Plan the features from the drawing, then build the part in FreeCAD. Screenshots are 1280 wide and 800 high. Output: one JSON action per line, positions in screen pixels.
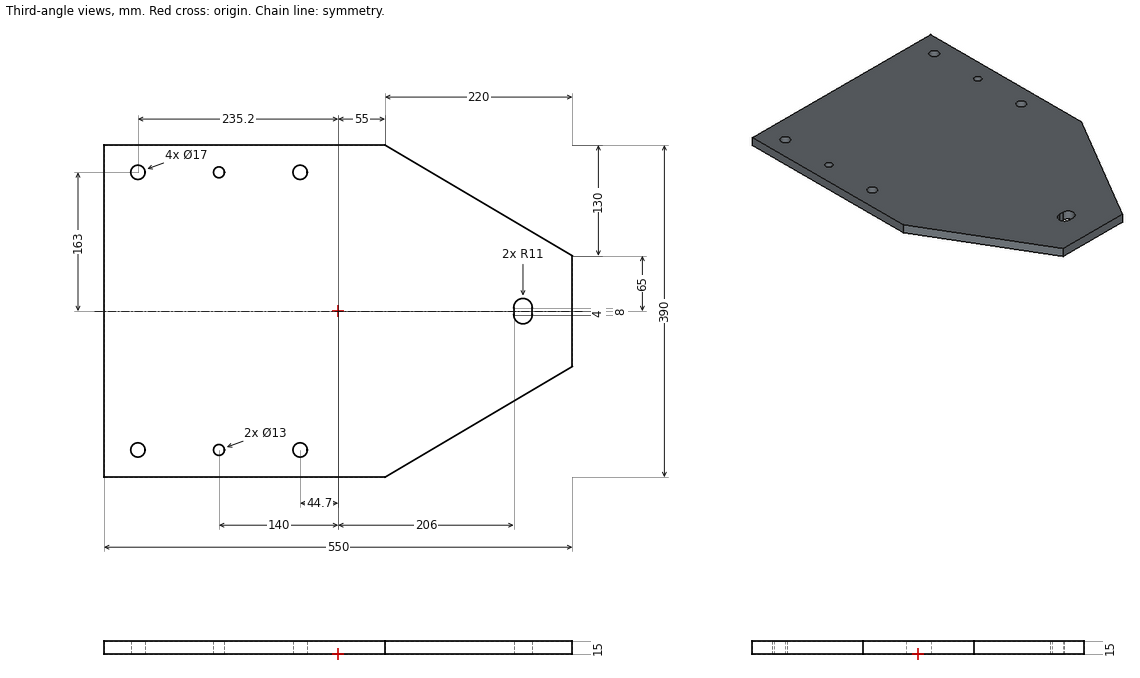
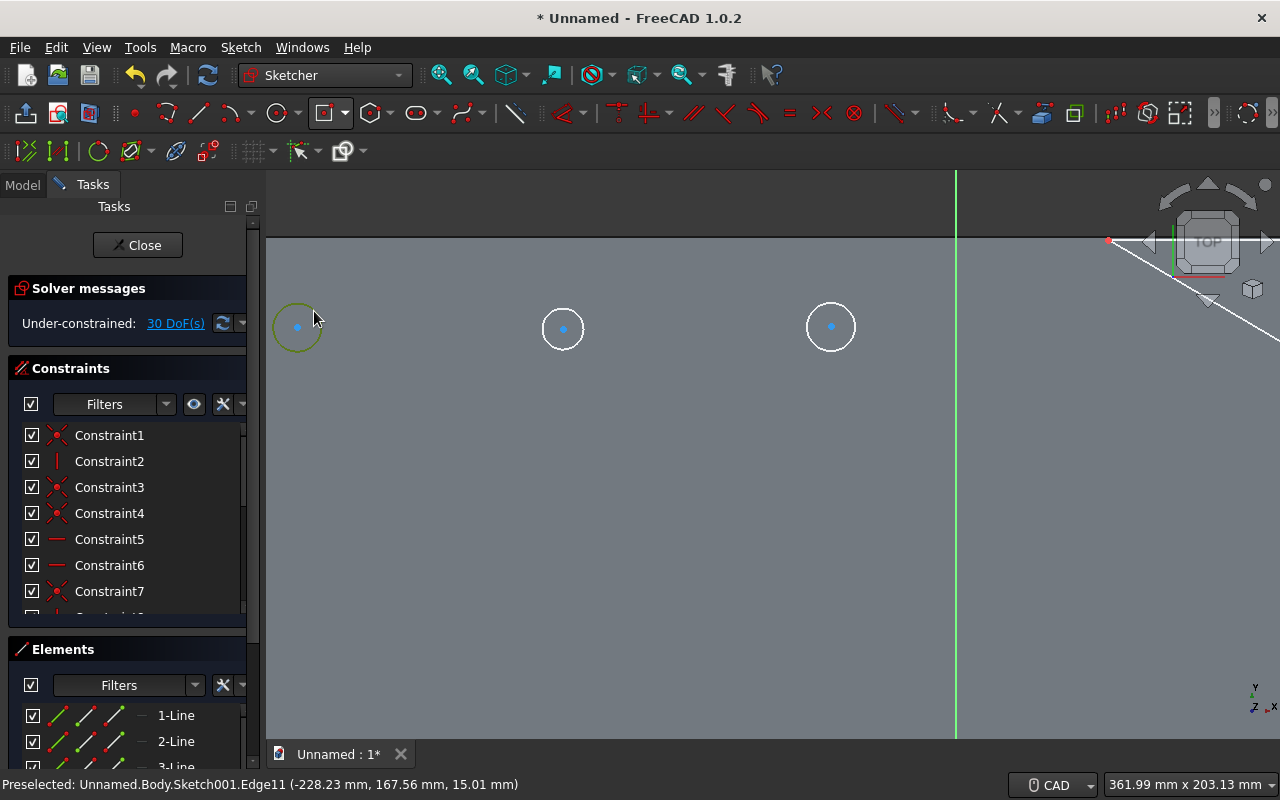
{"action": "scroll", "coordinate": [577, 313], "scroll_direction": "down", "scroll_amount": 6}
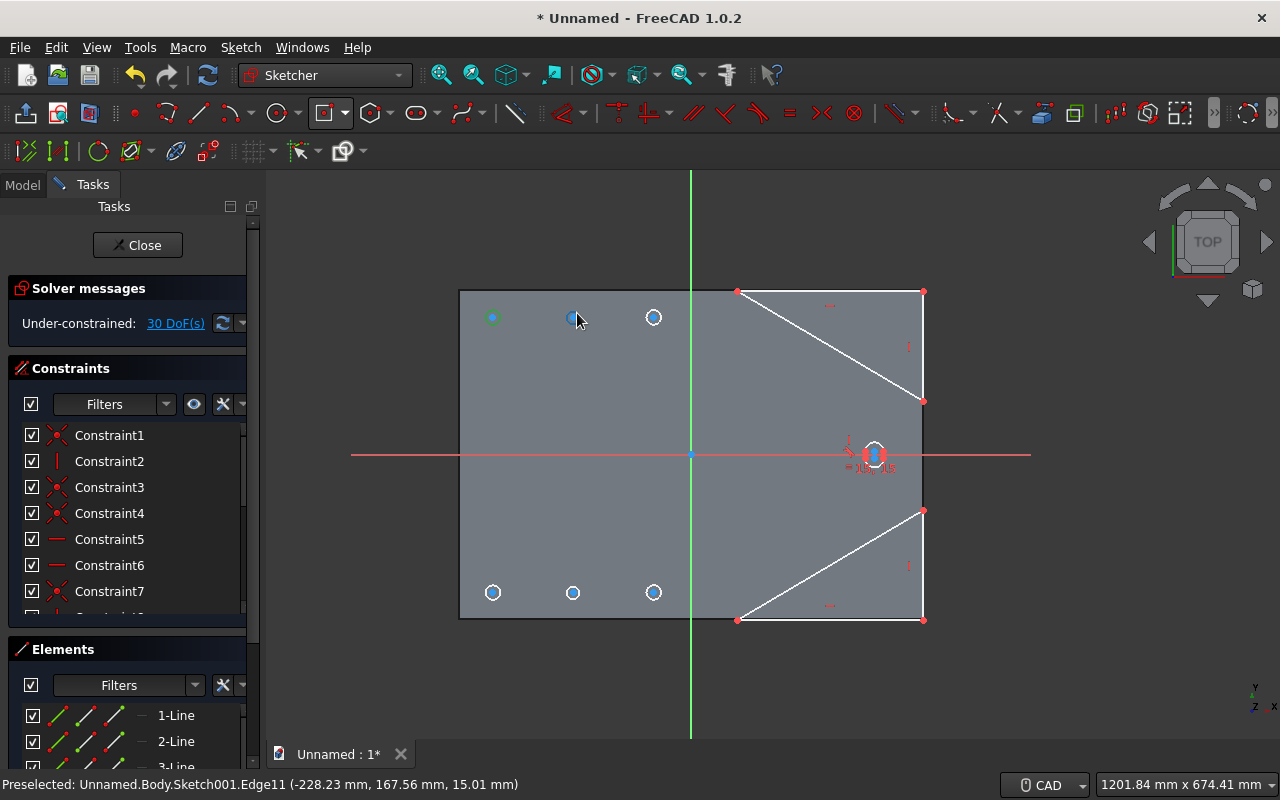
{"action": "scroll", "coordinate": [498, 587], "scroll_direction": "up", "scroll_amount": 4}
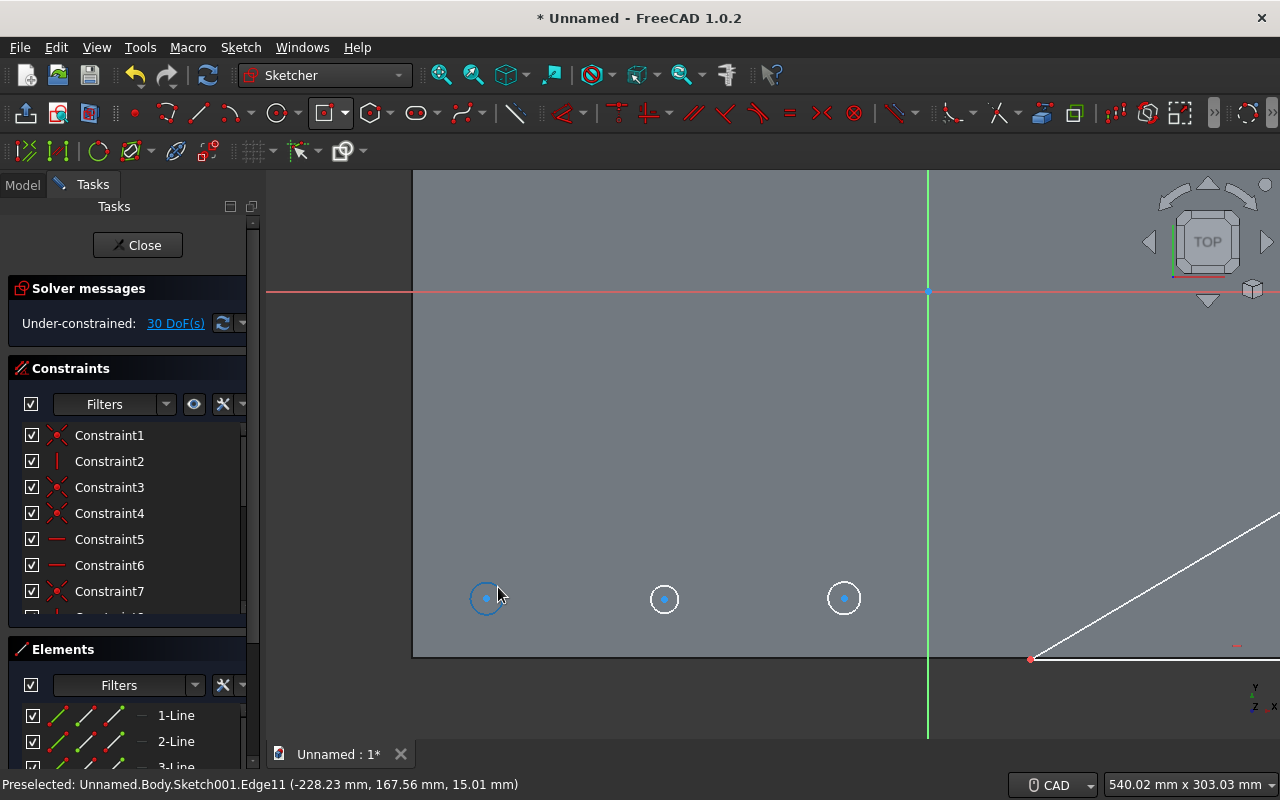
{"action": "left_click", "coordinate": [498, 587]}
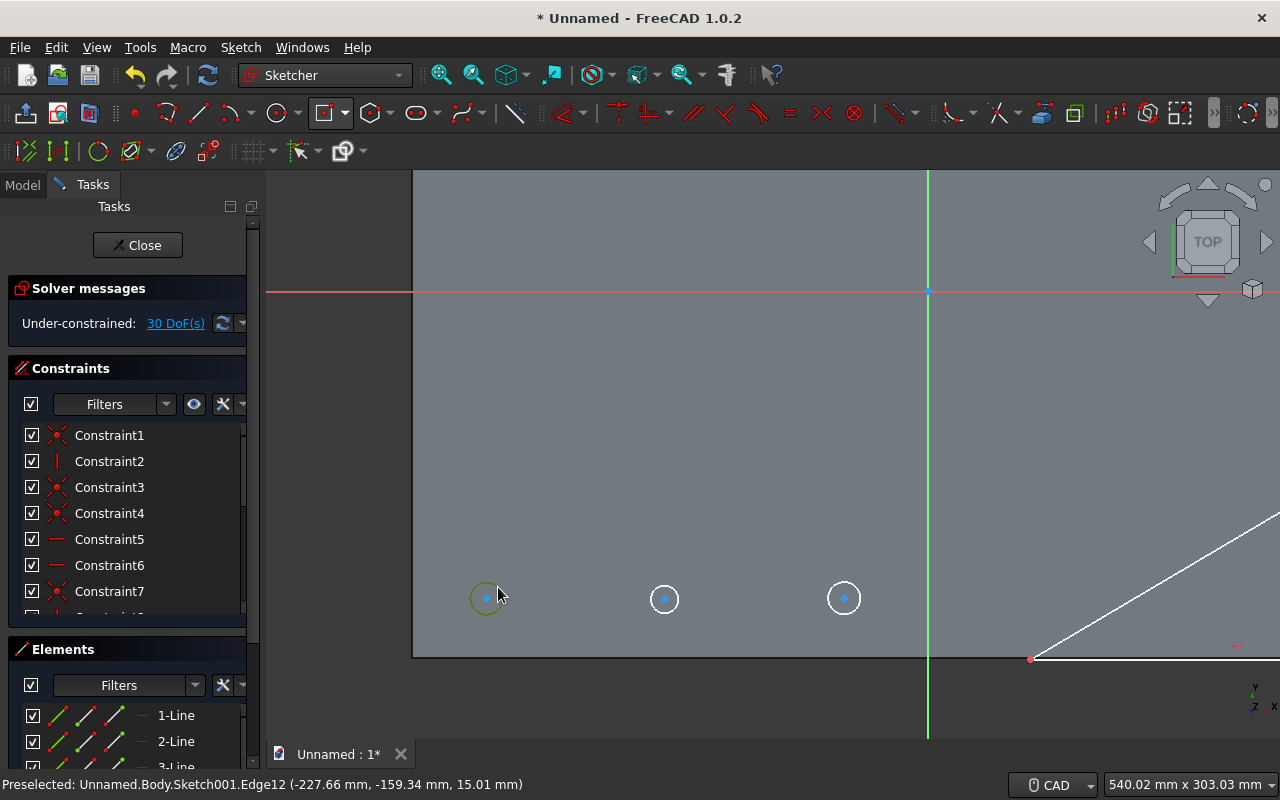
{"action": "left_click", "coordinate": [856, 587]}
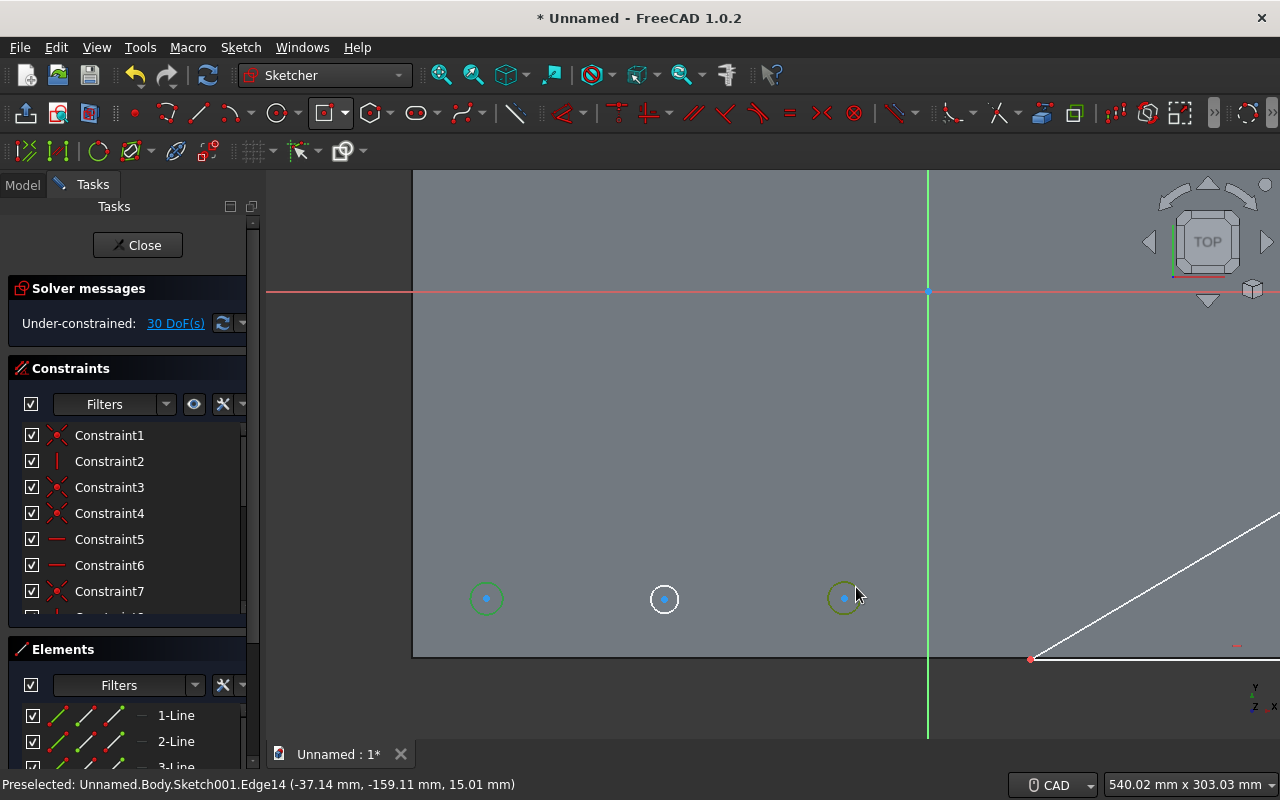
{"action": "scroll", "coordinate": [498, 587], "scroll_direction": "down", "scroll_amount": 4}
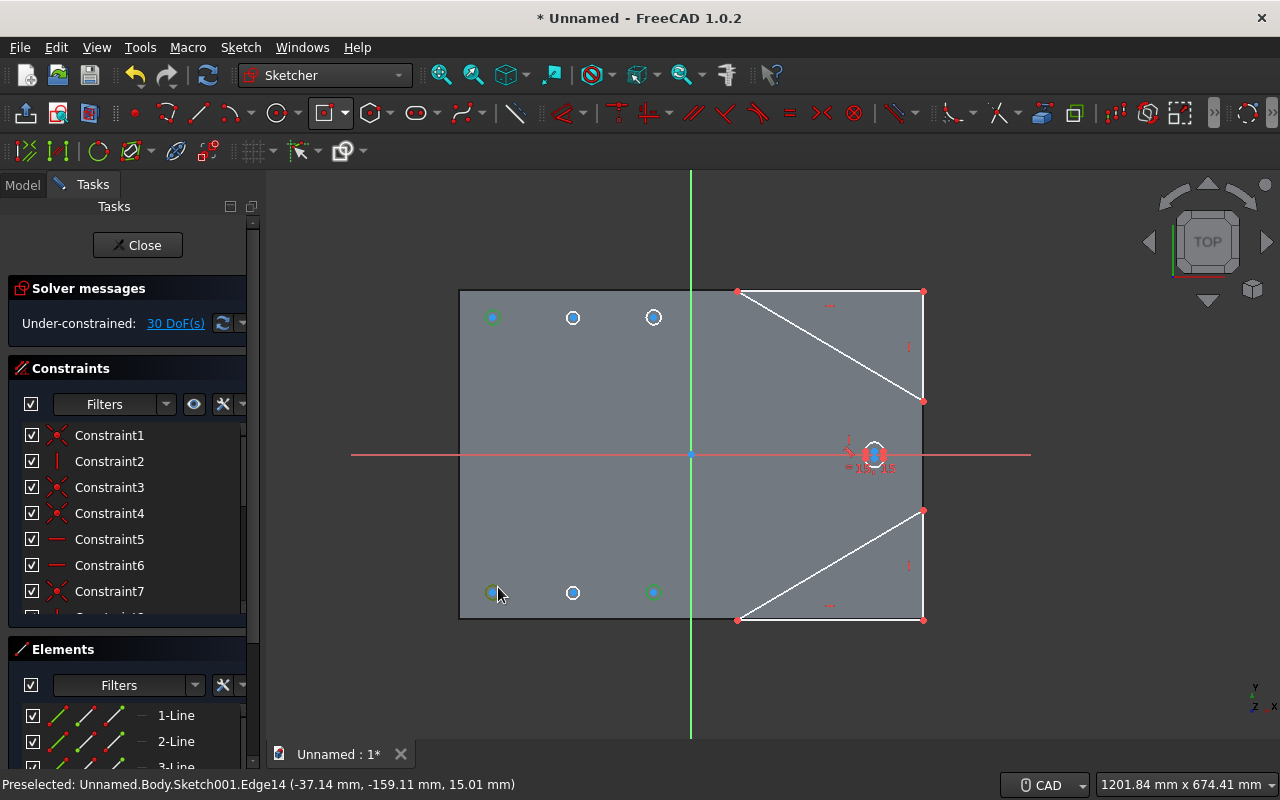
{"action": "scroll", "coordinate": [659, 312], "scroll_direction": "up", "scroll_amount": 4}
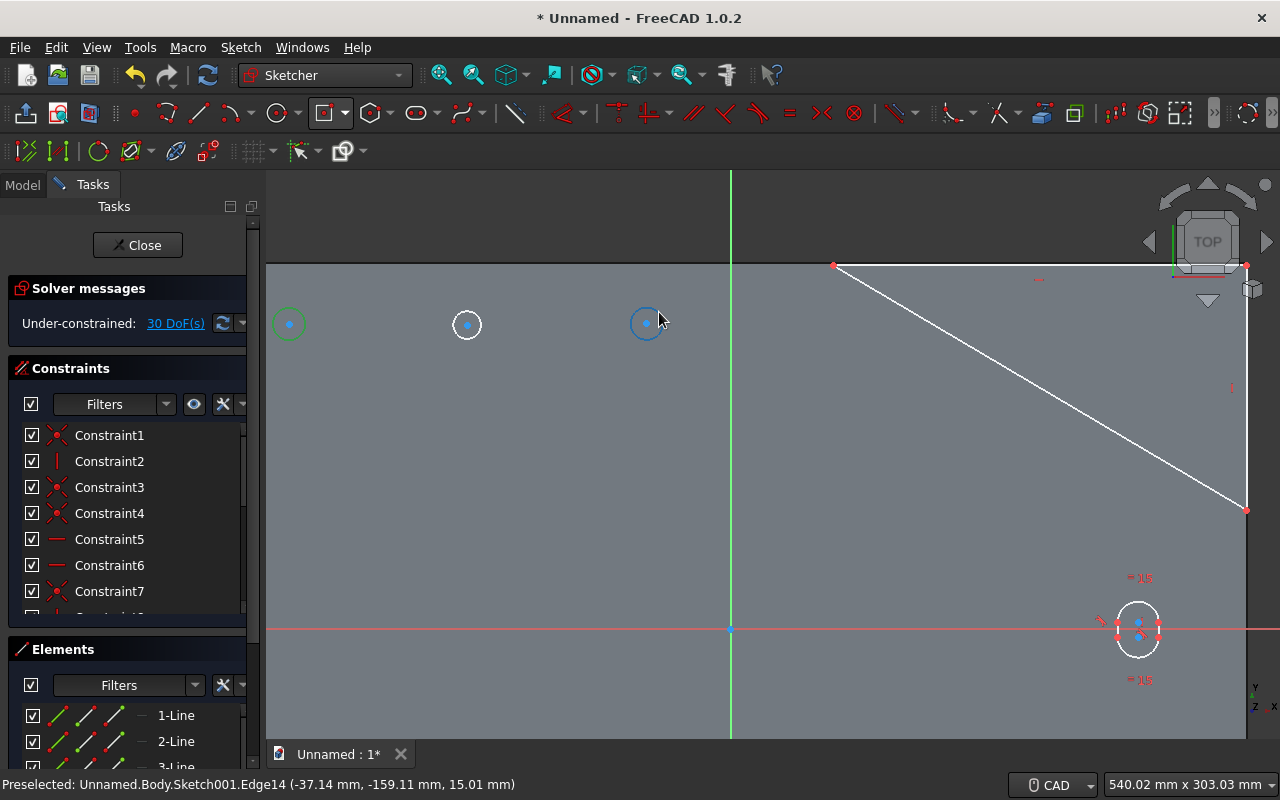
{"action": "left_click", "coordinate": [658, 312]}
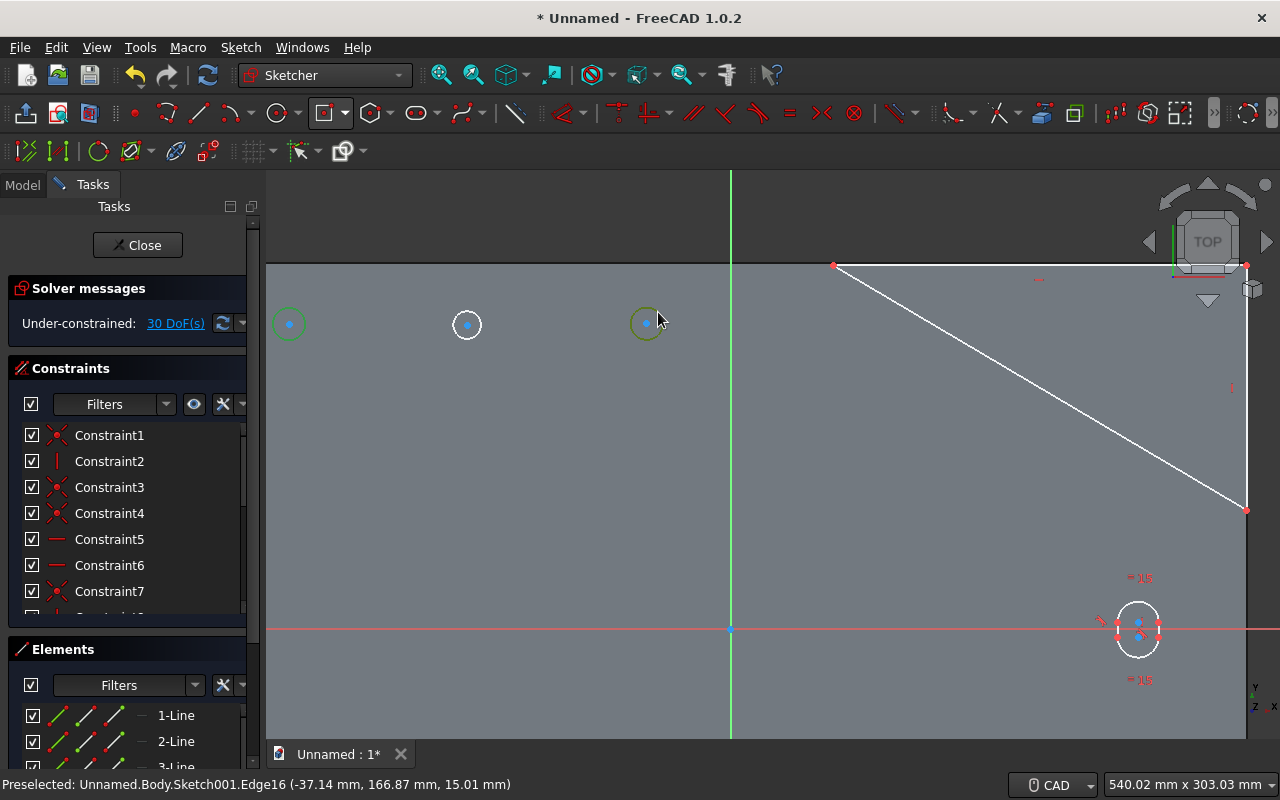
{"action": "left_click", "coordinate": [790, 114]}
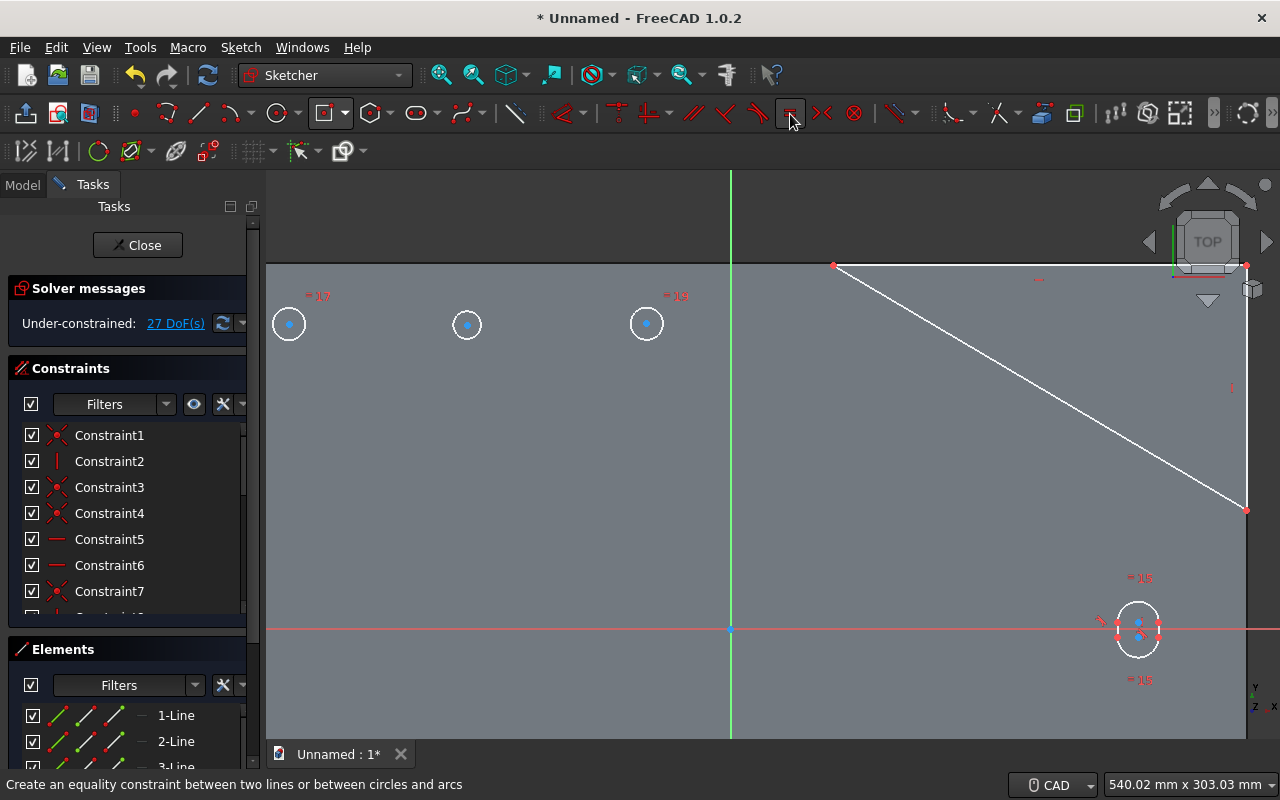
{"action": "scroll", "coordinate": [659, 312], "scroll_direction": "down", "scroll_amount": 4}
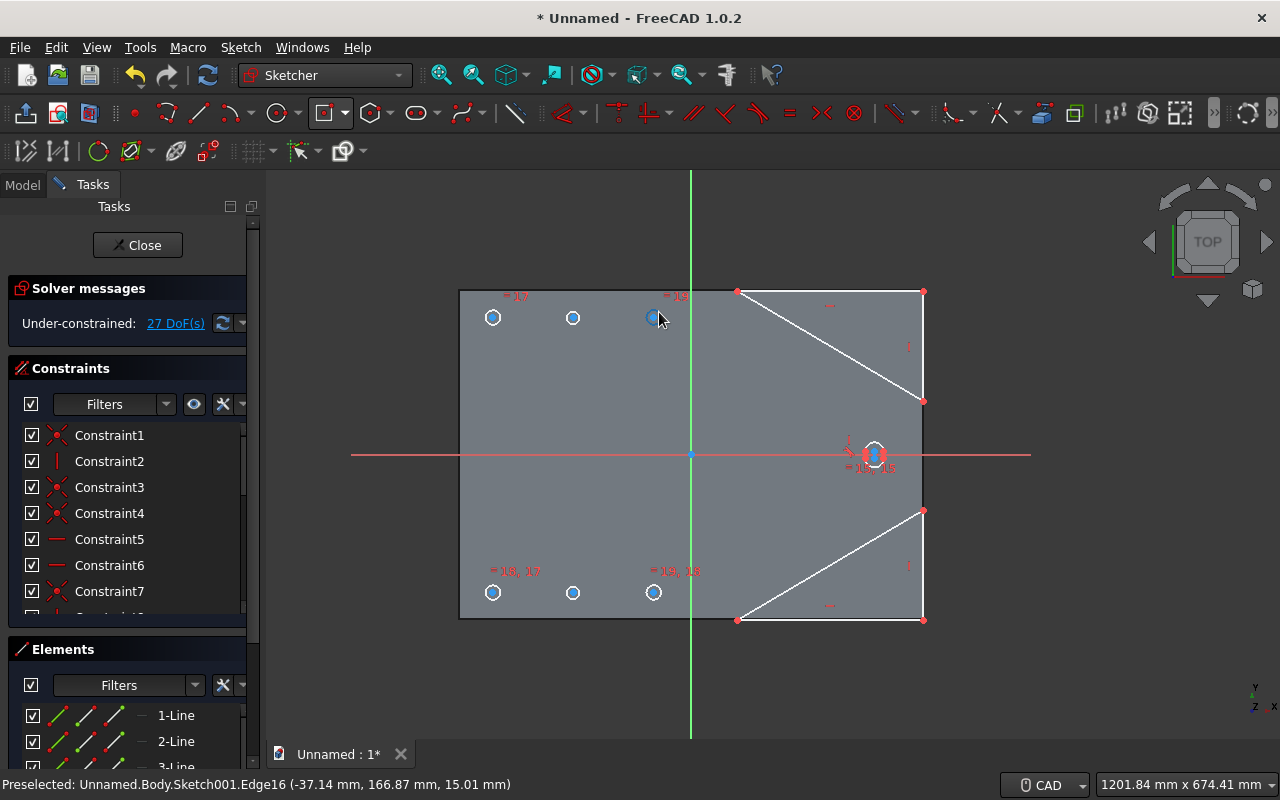
{"action": "scroll", "coordinate": [577, 589], "scroll_direction": "up", "scroll_amount": 5}